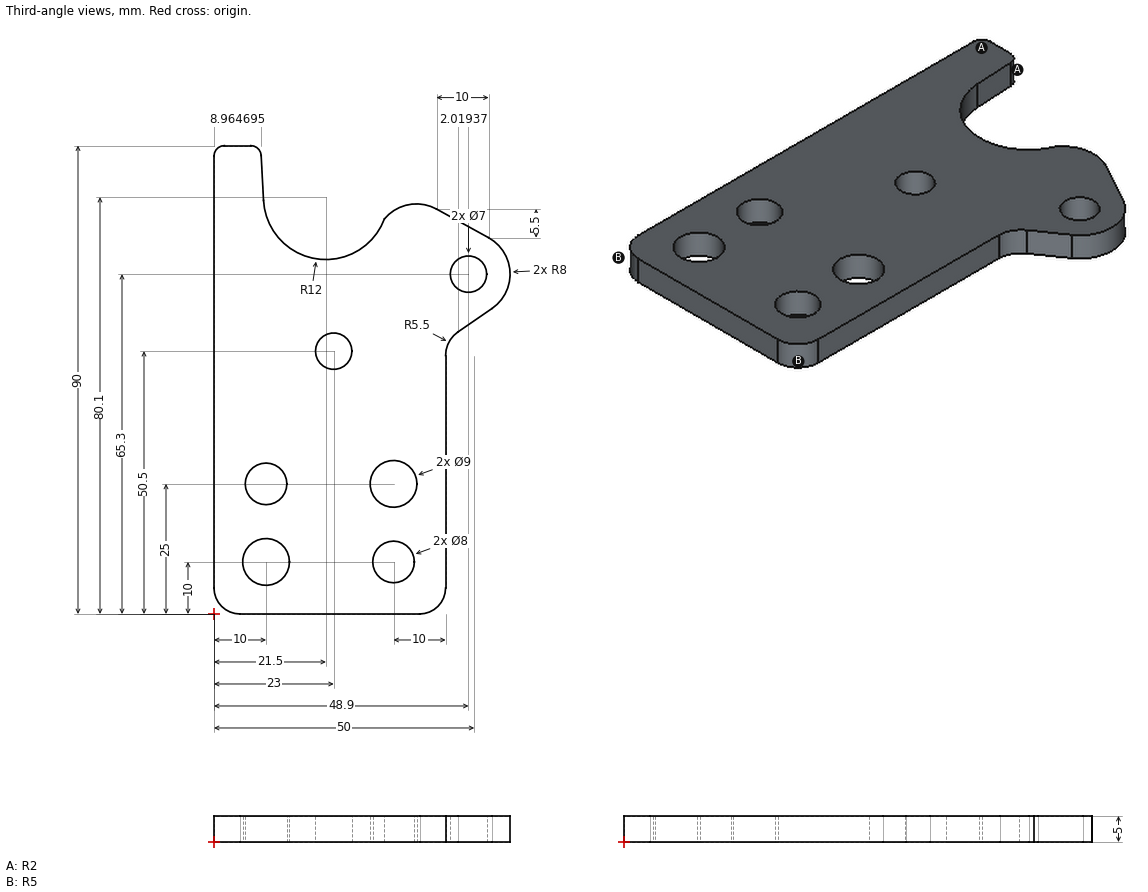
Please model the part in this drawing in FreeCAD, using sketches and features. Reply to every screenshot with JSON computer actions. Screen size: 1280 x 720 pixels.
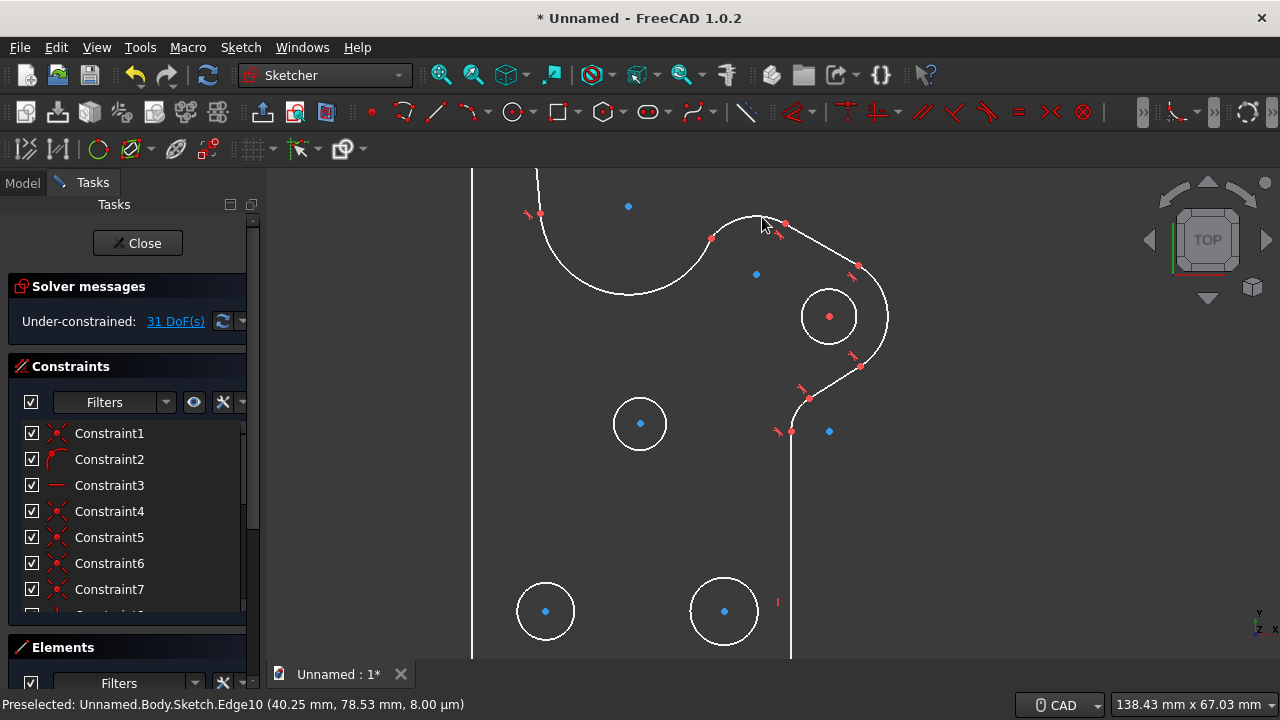
{"action": "scroll", "coordinate": [724, 373], "scroll_direction": "down", "scroll_amount": 4}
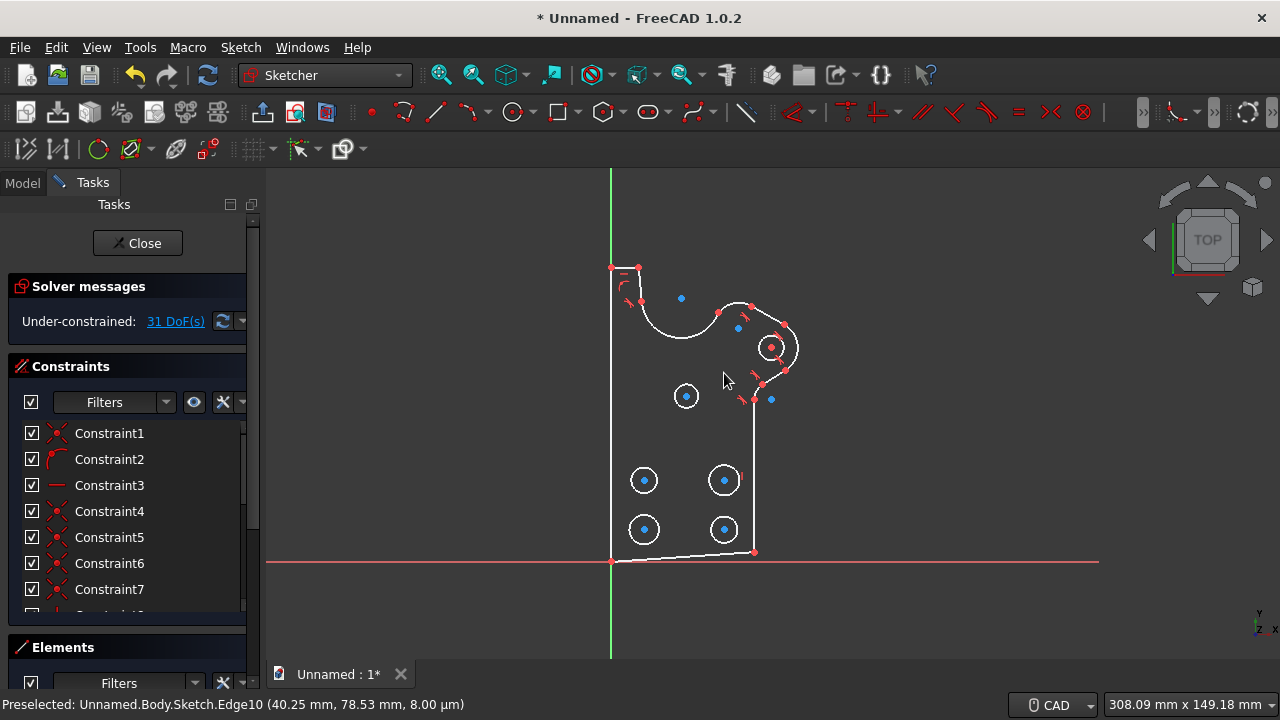
{"action": "scroll", "coordinate": [711, 555], "scroll_direction": "up", "scroll_amount": 4}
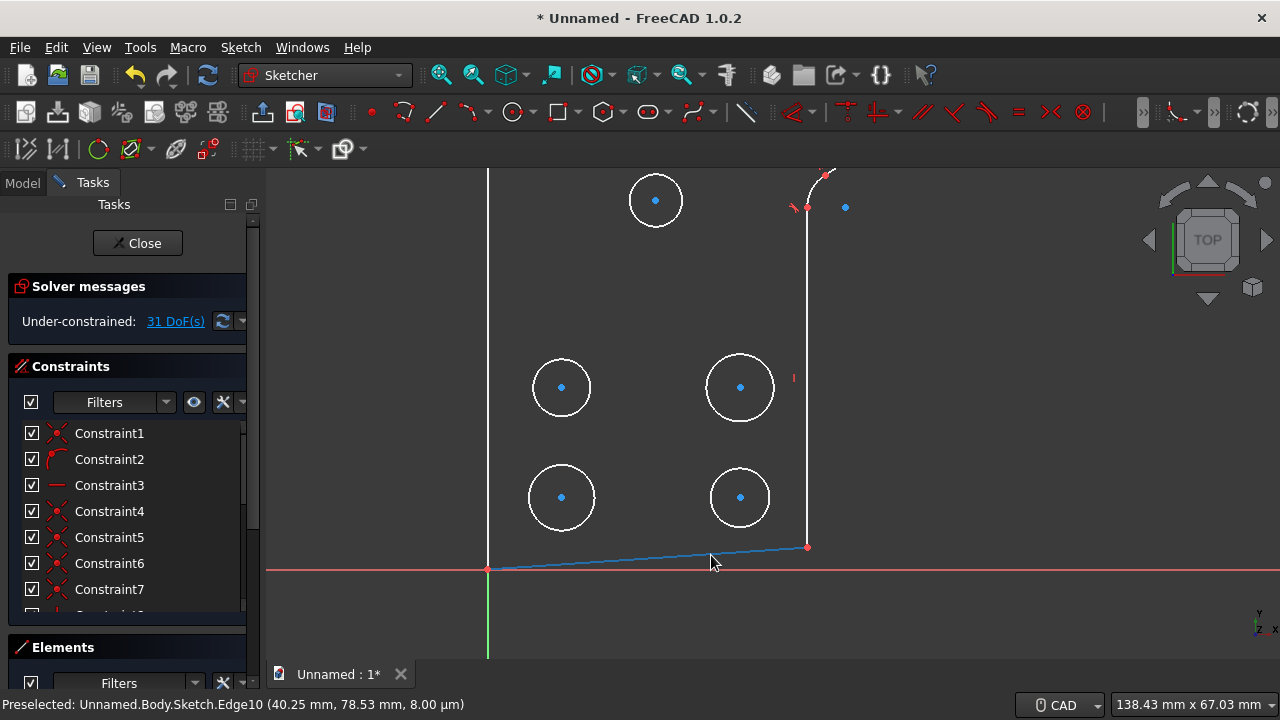
{"action": "left_click", "coordinate": [711, 554]}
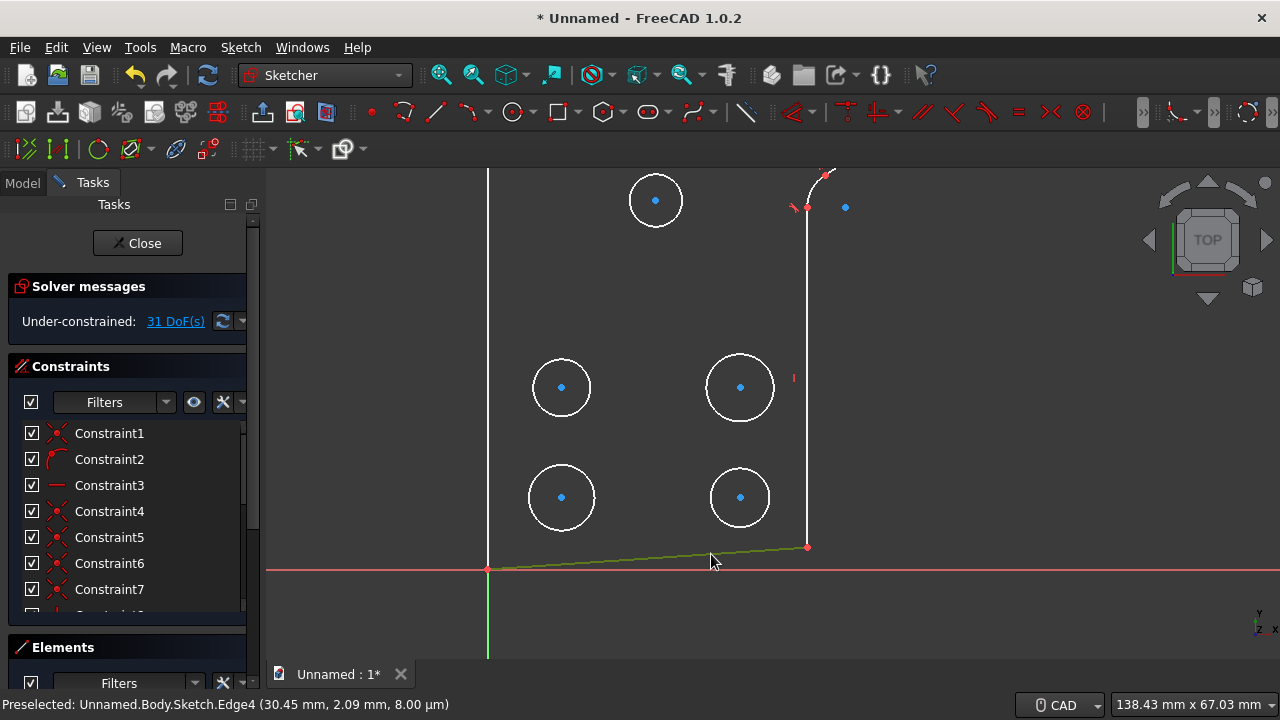
{"action": "key", "text": "h"}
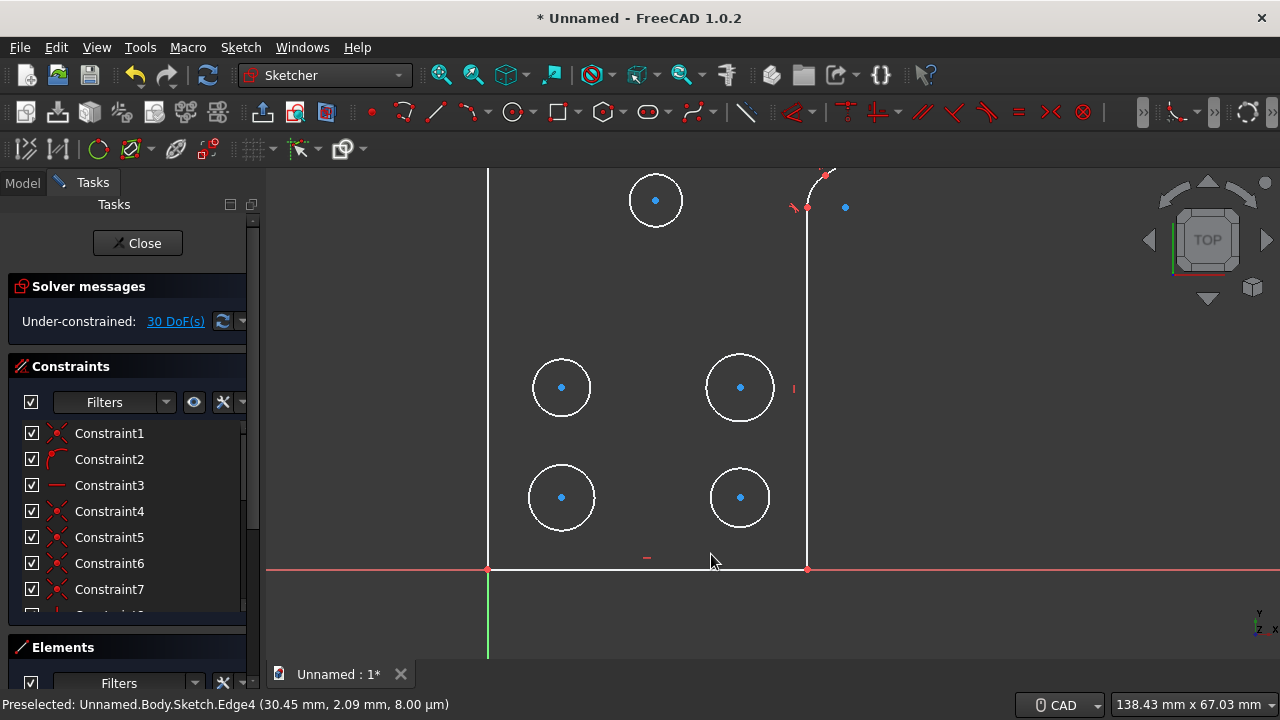
{"action": "scroll", "coordinate": [711, 555], "scroll_direction": "down", "scroll_amount": 4}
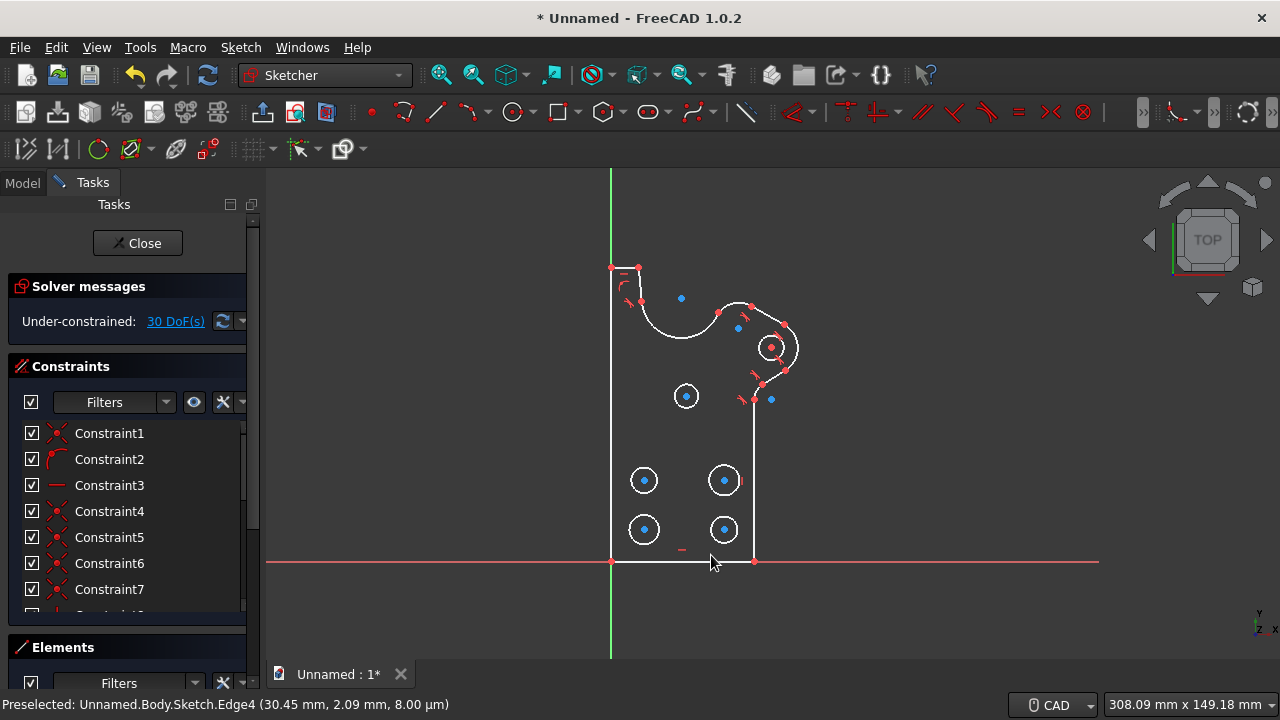
{"action": "left_click", "coordinate": [796, 358]}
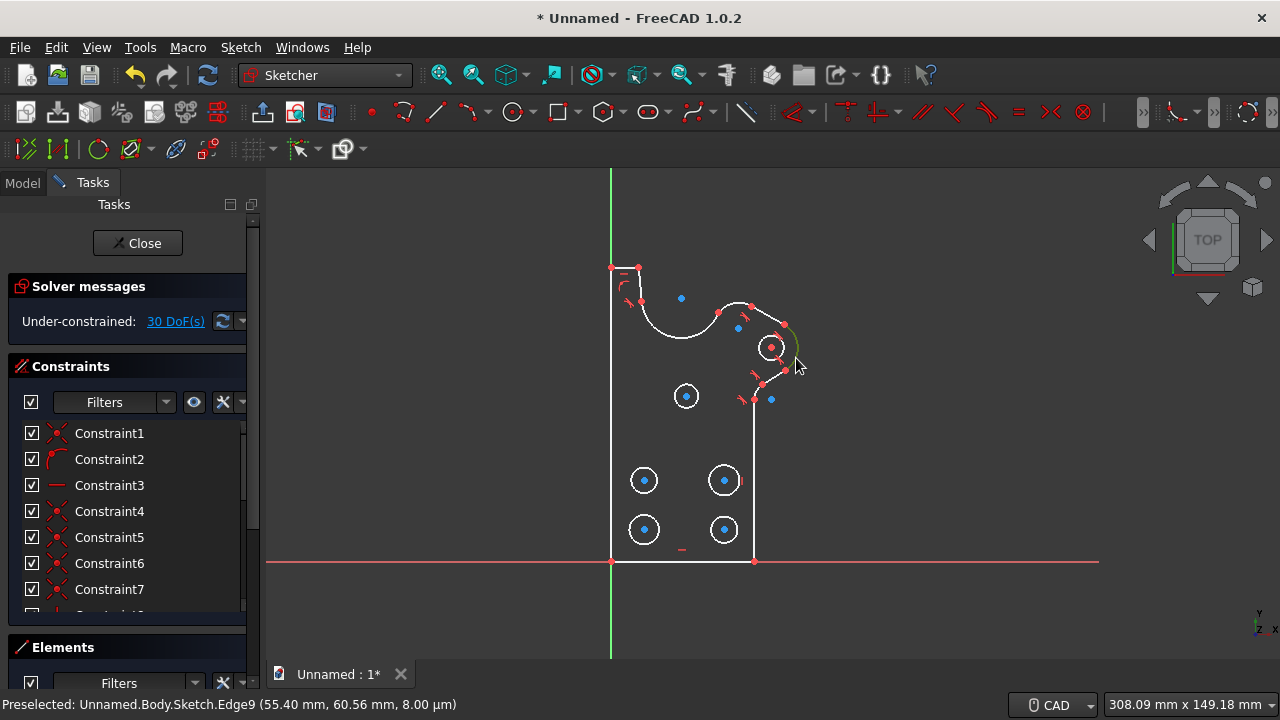
{"action": "scroll", "coordinate": [741, 303], "scroll_direction": "up", "scroll_amount": 2}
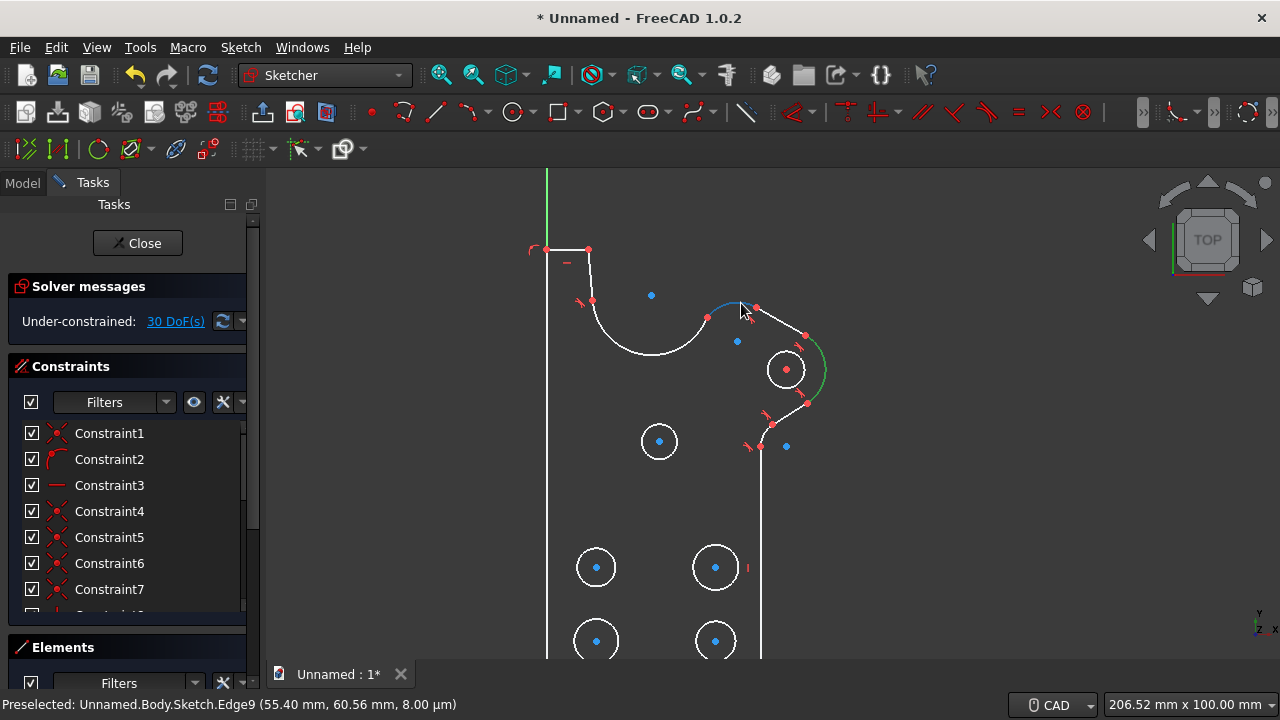
{"action": "left_click", "coordinate": [741, 303]}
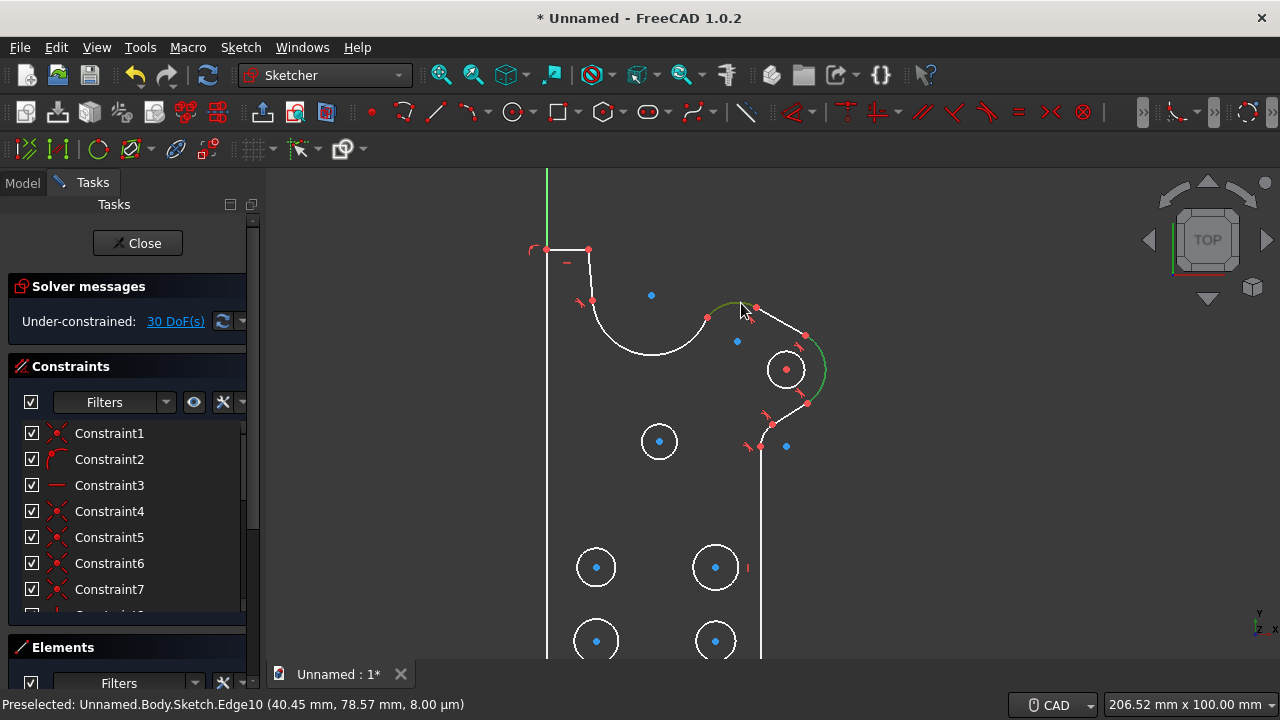
{"action": "key", "text": "e"}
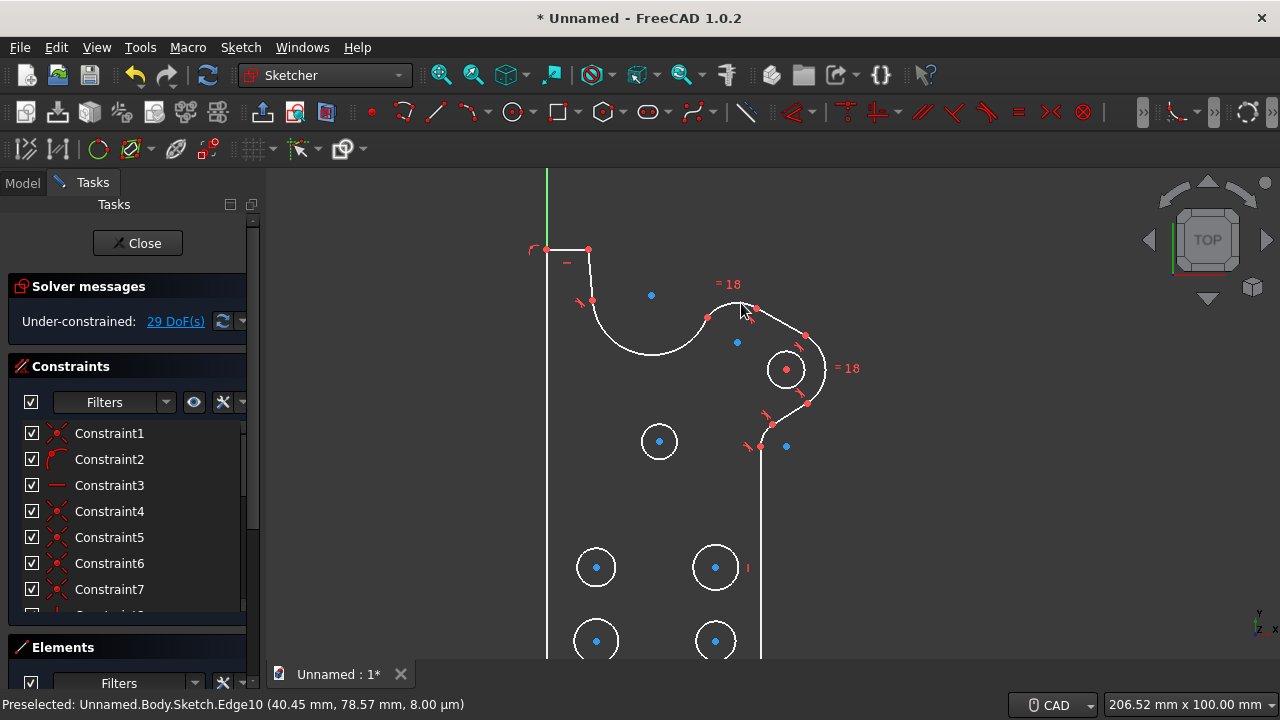
{"action": "left_click", "coordinate": [732, 551]}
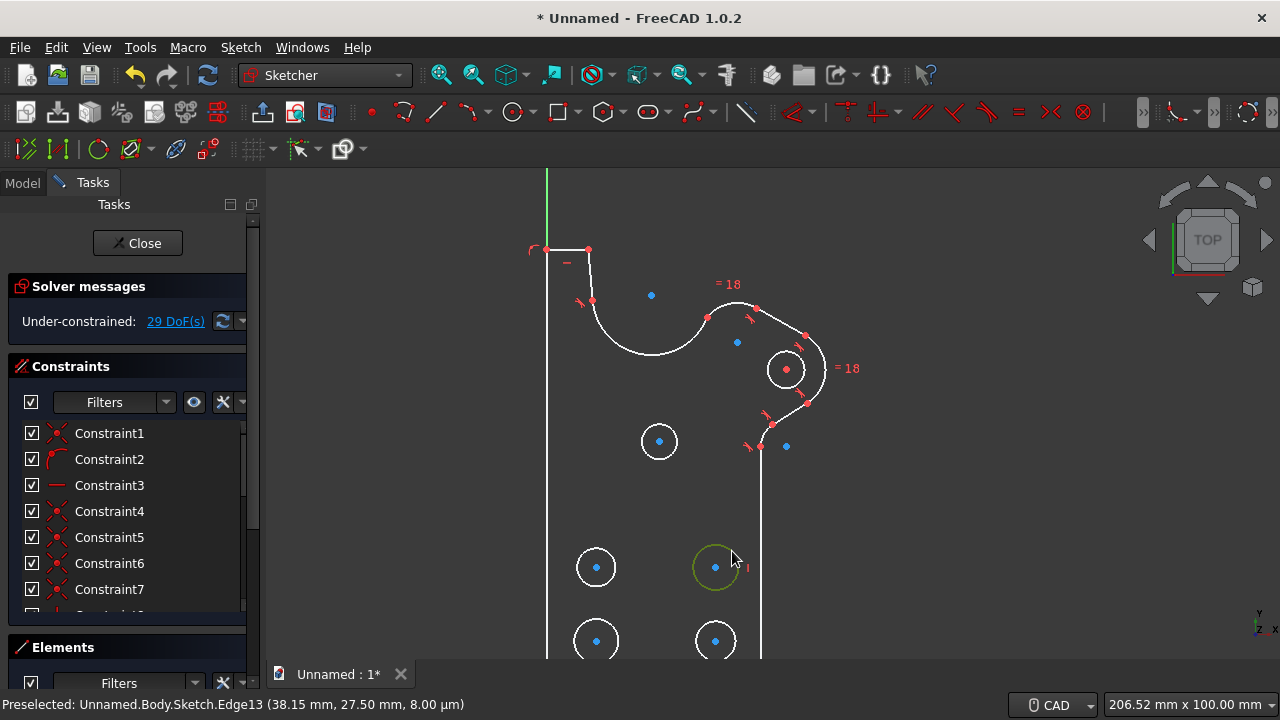
{"action": "left_click", "coordinate": [612, 625]}